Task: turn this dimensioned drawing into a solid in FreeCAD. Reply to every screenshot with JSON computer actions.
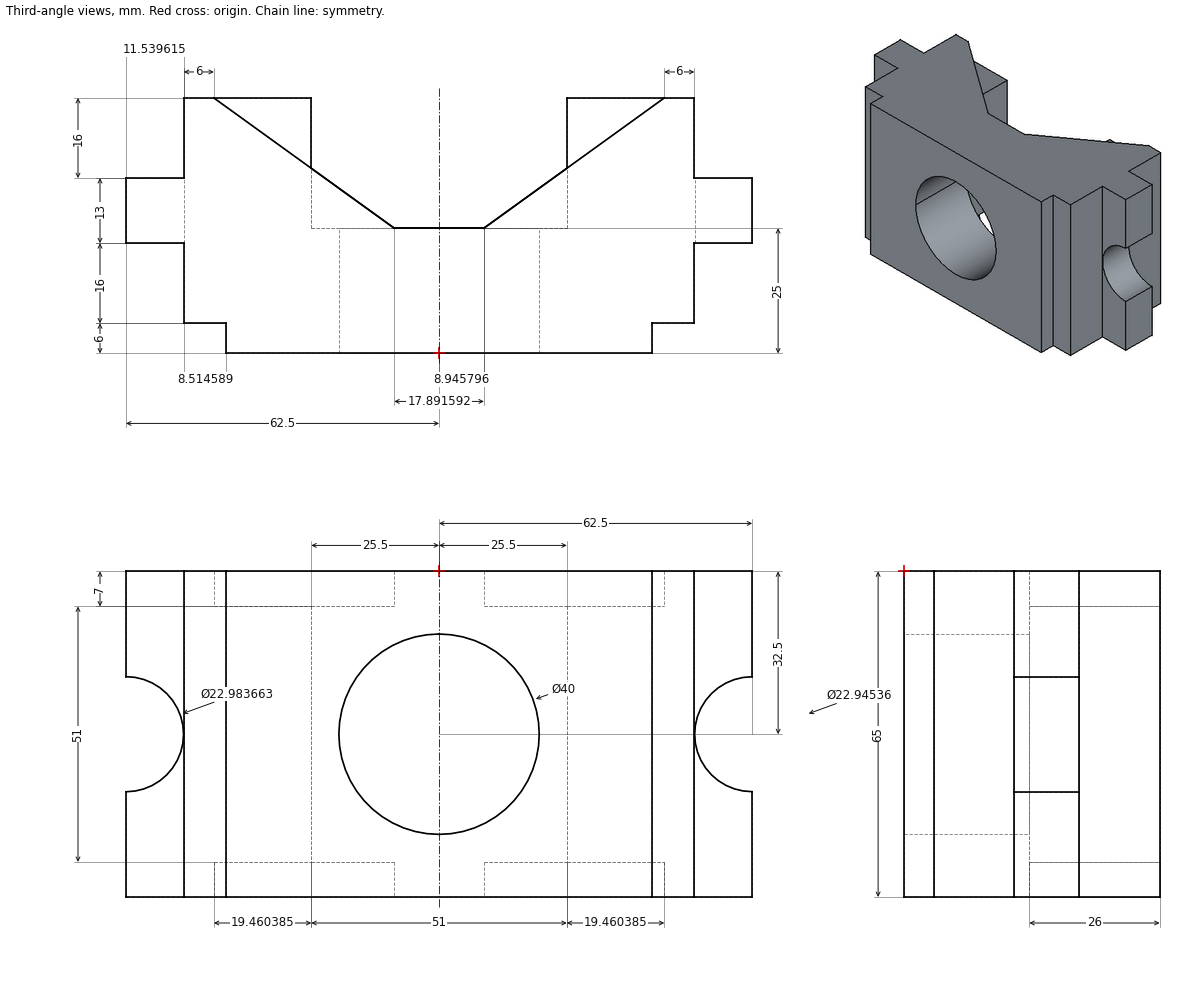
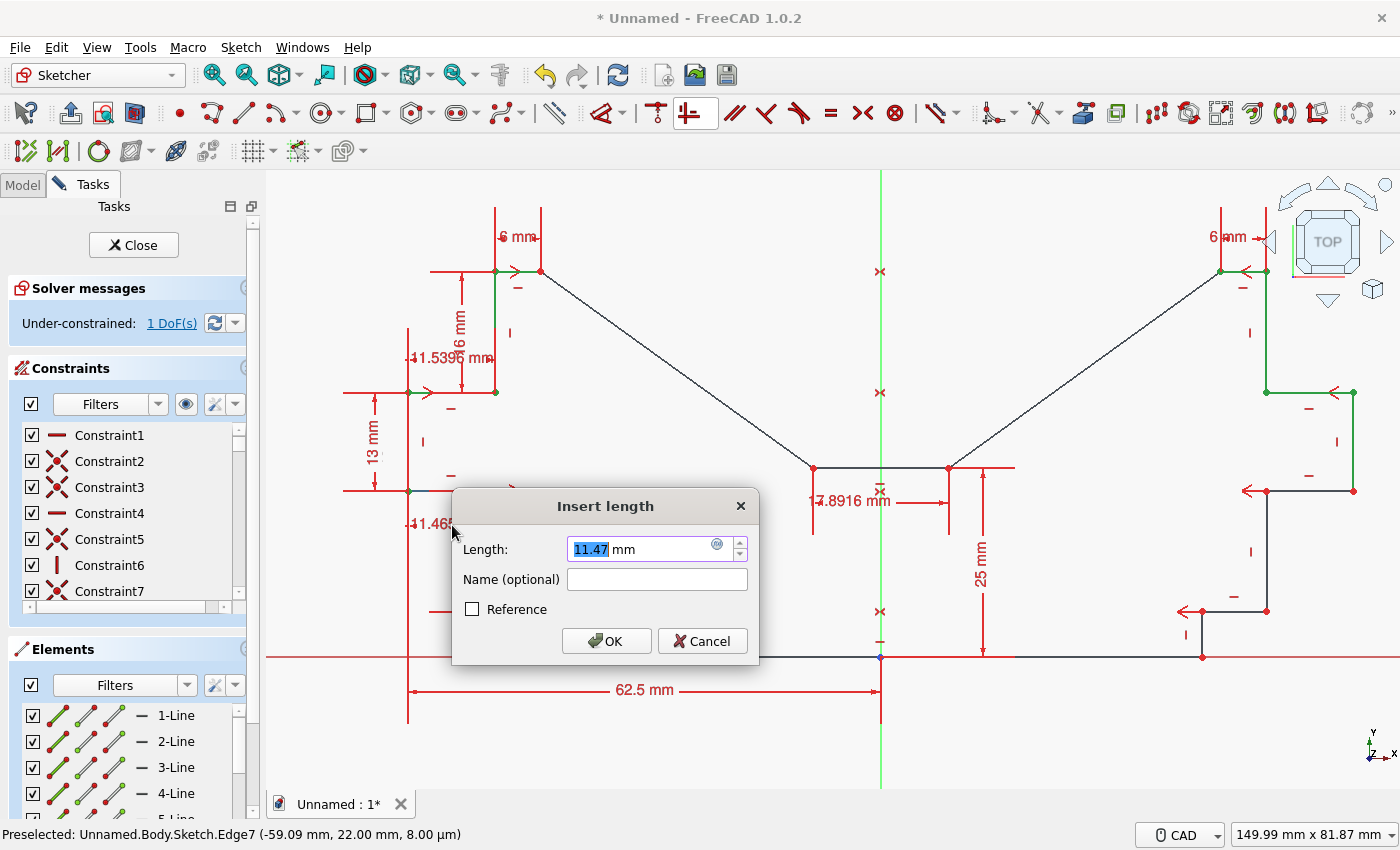
{"action": "type", "text": "11.539615"}
{"action": "key", "text": "Return"}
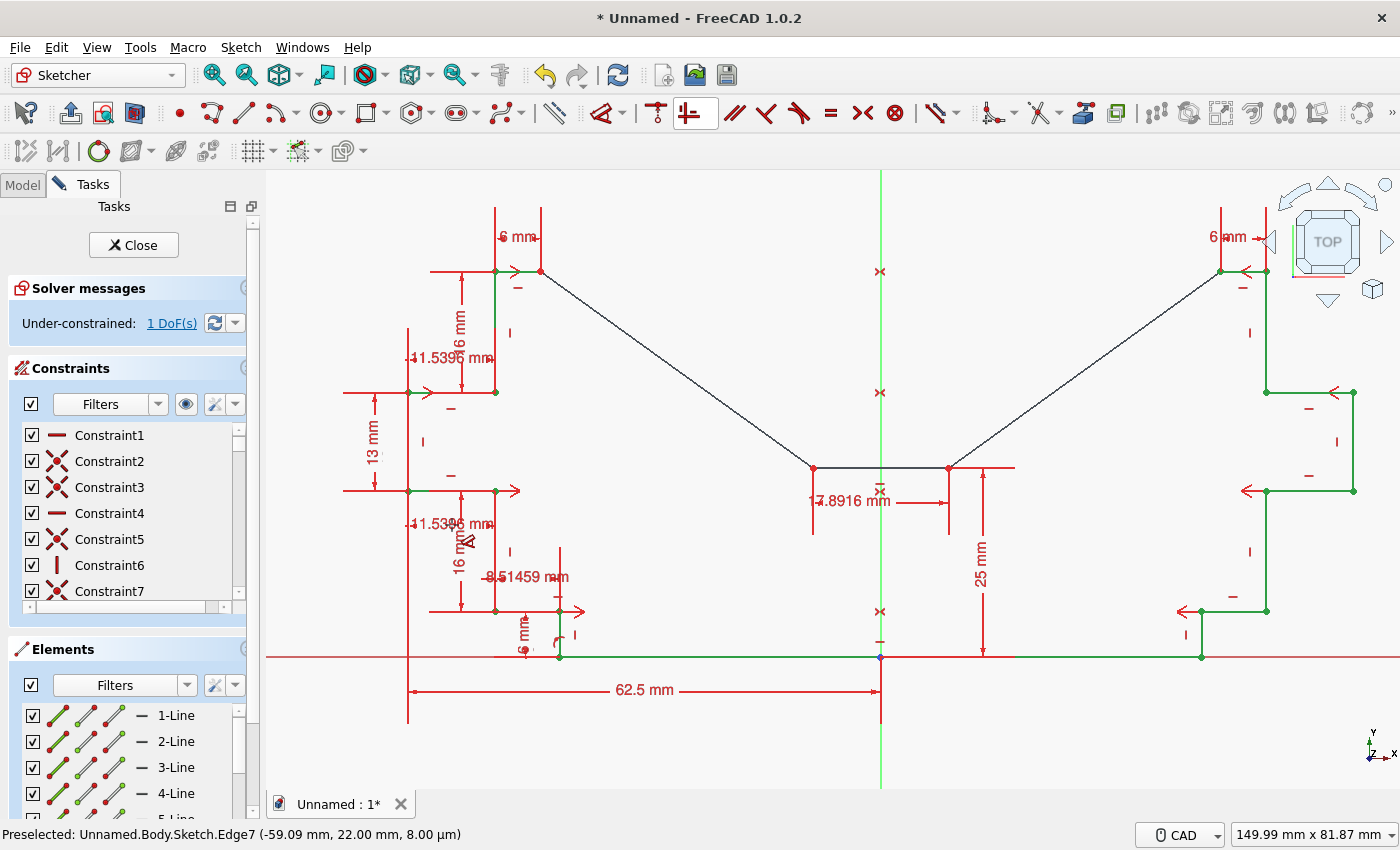
{"action": "left_click", "coordinate": [949, 468]}
{"action": "left_click", "coordinate": [915, 691]}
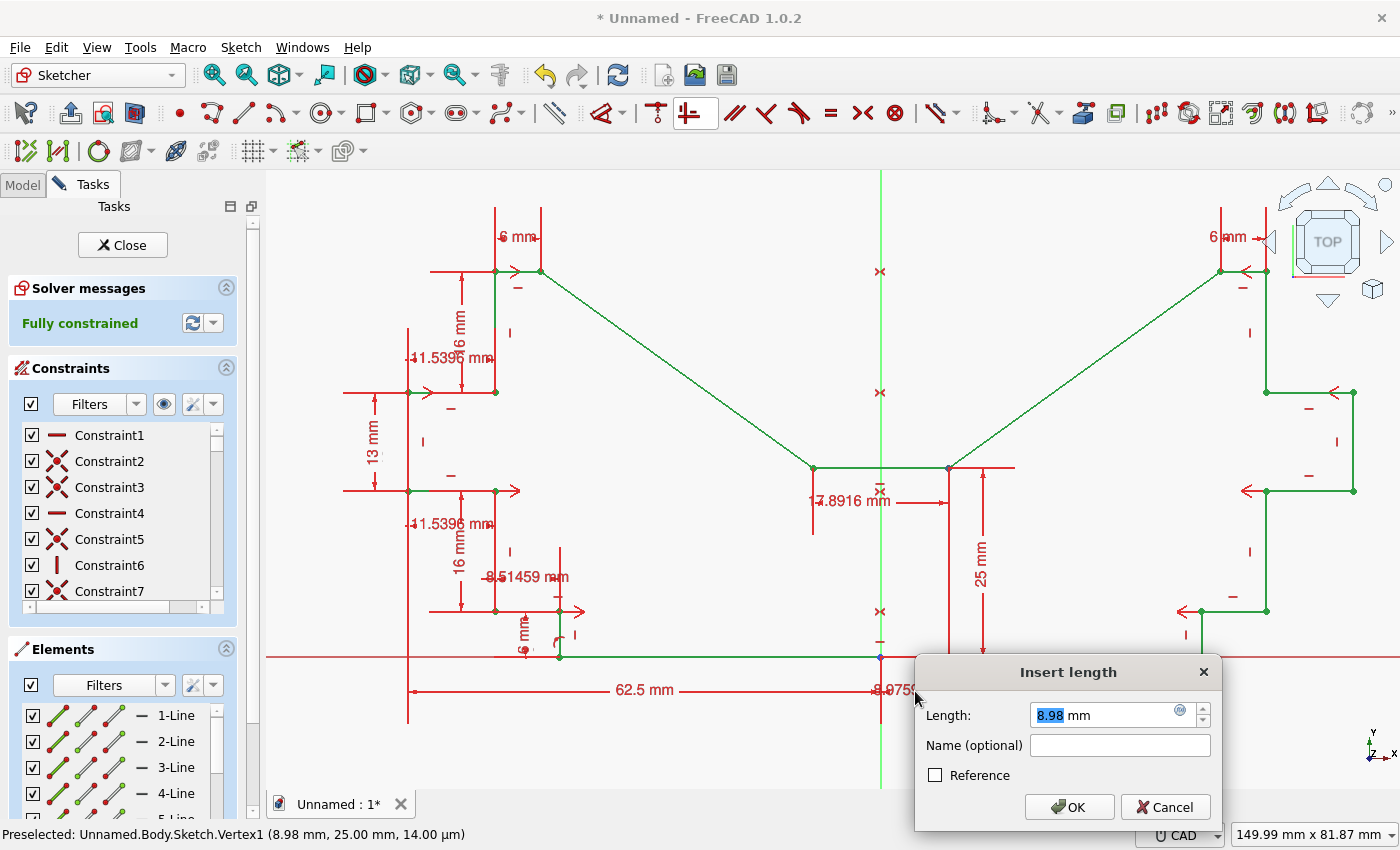
{"action": "type", "text": "8.945796"}
{"action": "key", "text": "Return"}
{"action": "key", "text": "Escape"}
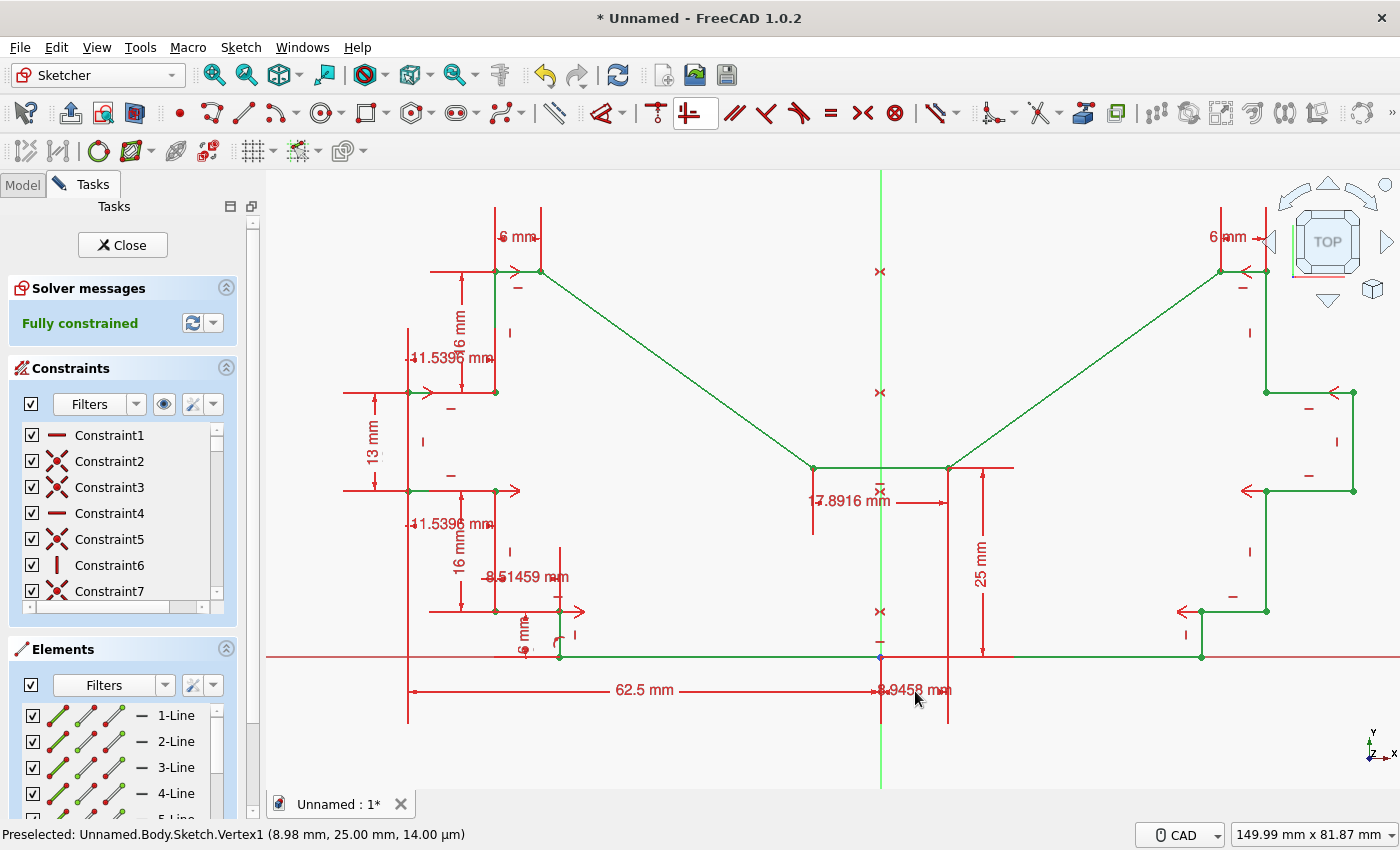
{"action": "left_click", "coordinate": [123, 245]}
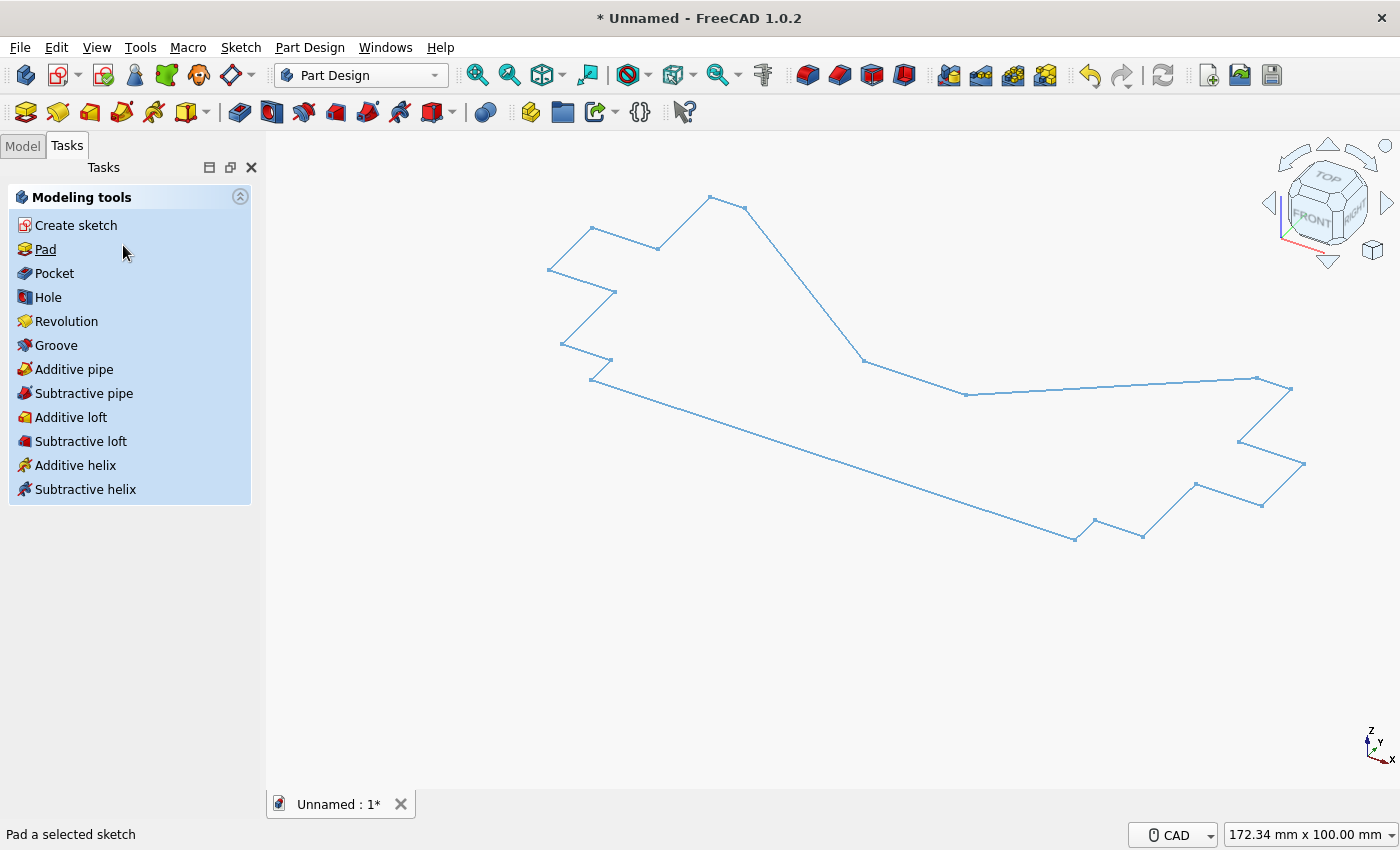
{"action": "left_click", "coordinate": [26, 112]}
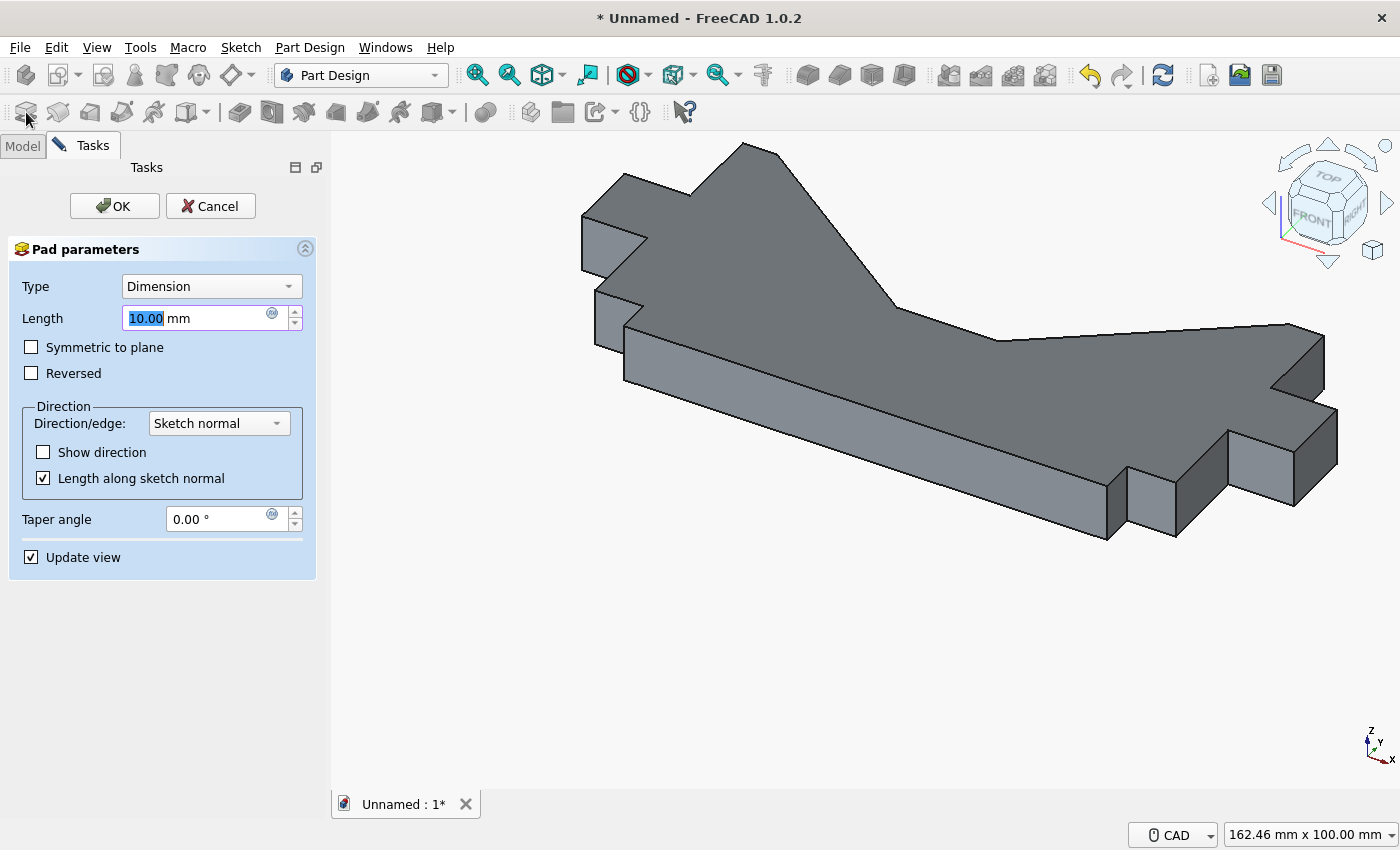
{"action": "type", "text": "65"}
{"action": "key", "text": "Tab"}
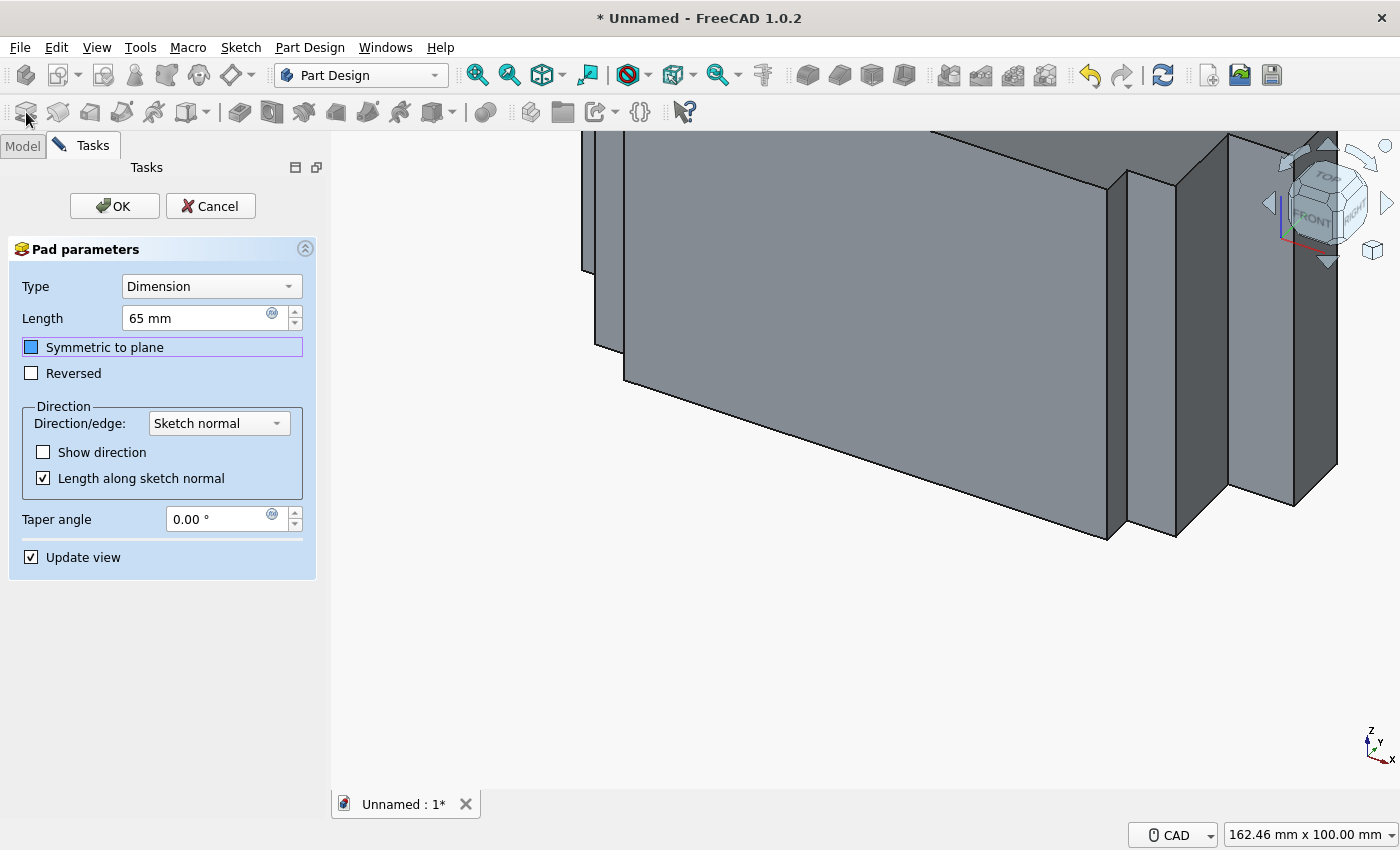
{"action": "left_click", "coordinate": [30, 373]}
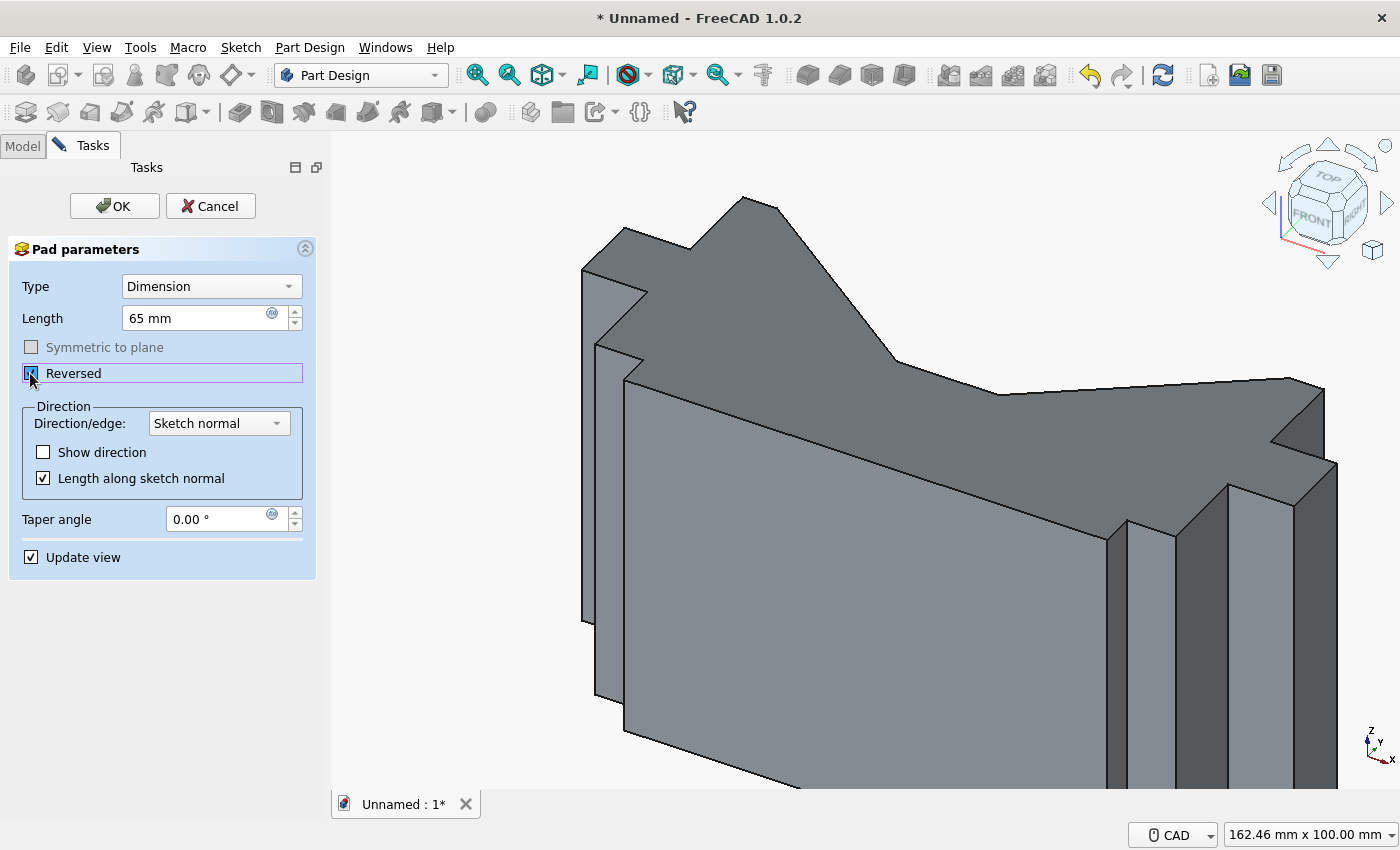
{"action": "left_click", "coordinate": [115, 206]}